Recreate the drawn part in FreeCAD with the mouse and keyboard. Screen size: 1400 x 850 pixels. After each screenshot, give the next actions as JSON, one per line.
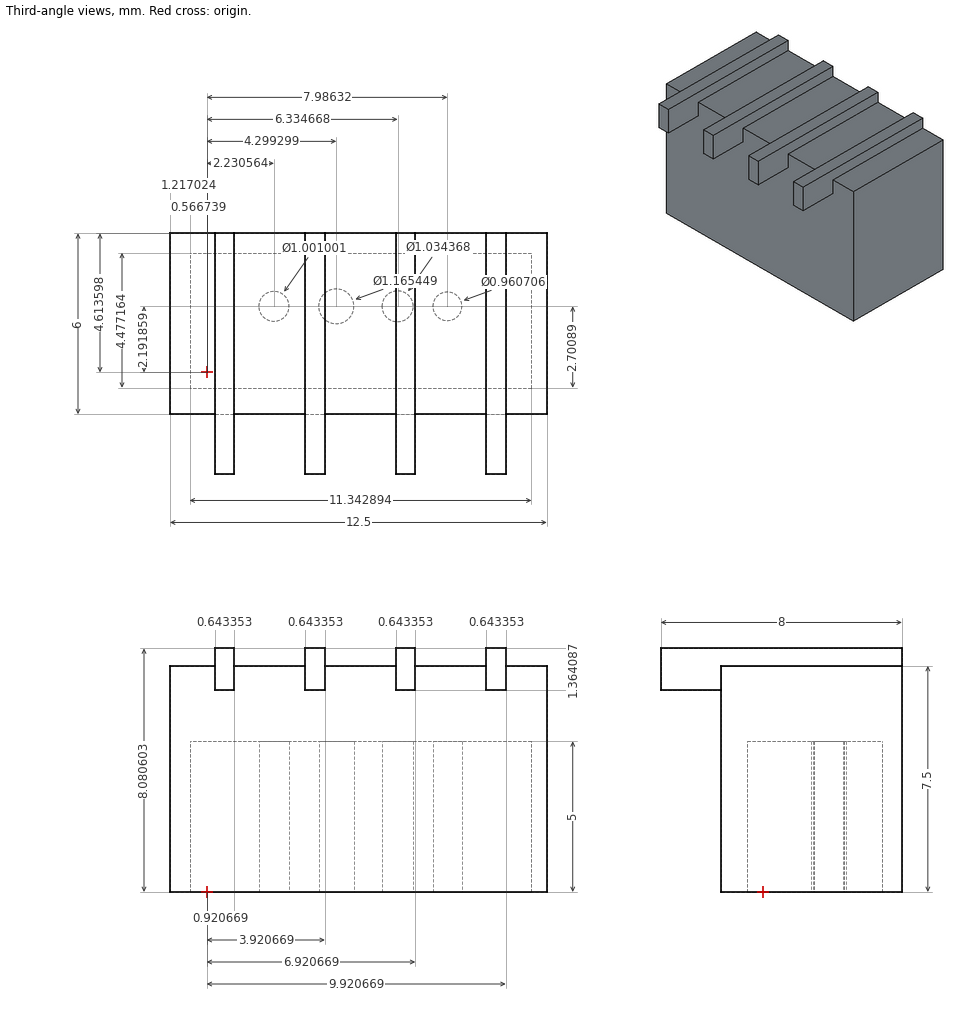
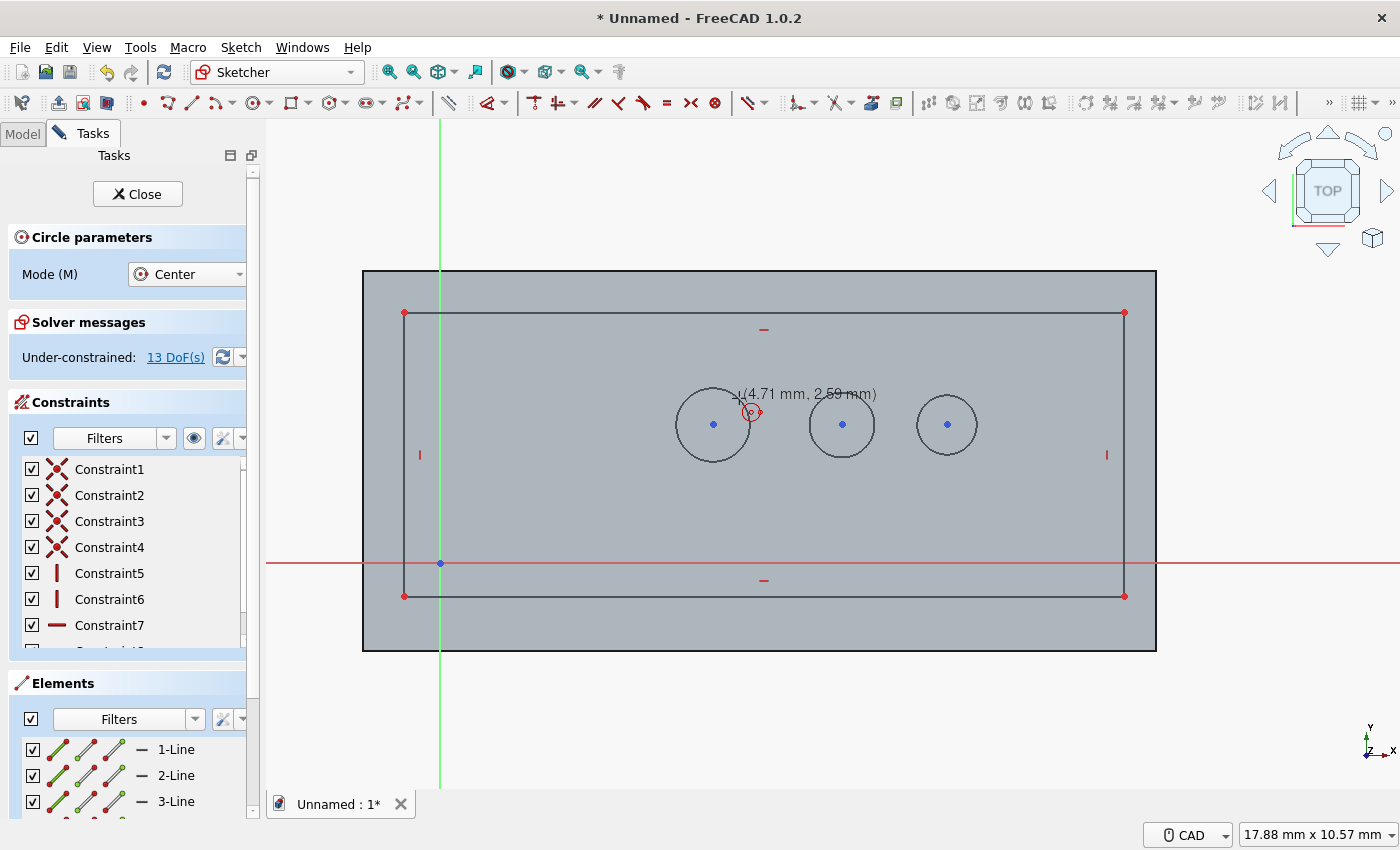
{"action": "left_click", "coordinate": [582, 424]}
{"action": "left_click", "coordinate": [604, 402]}
{"action": "key", "text": "Escape"}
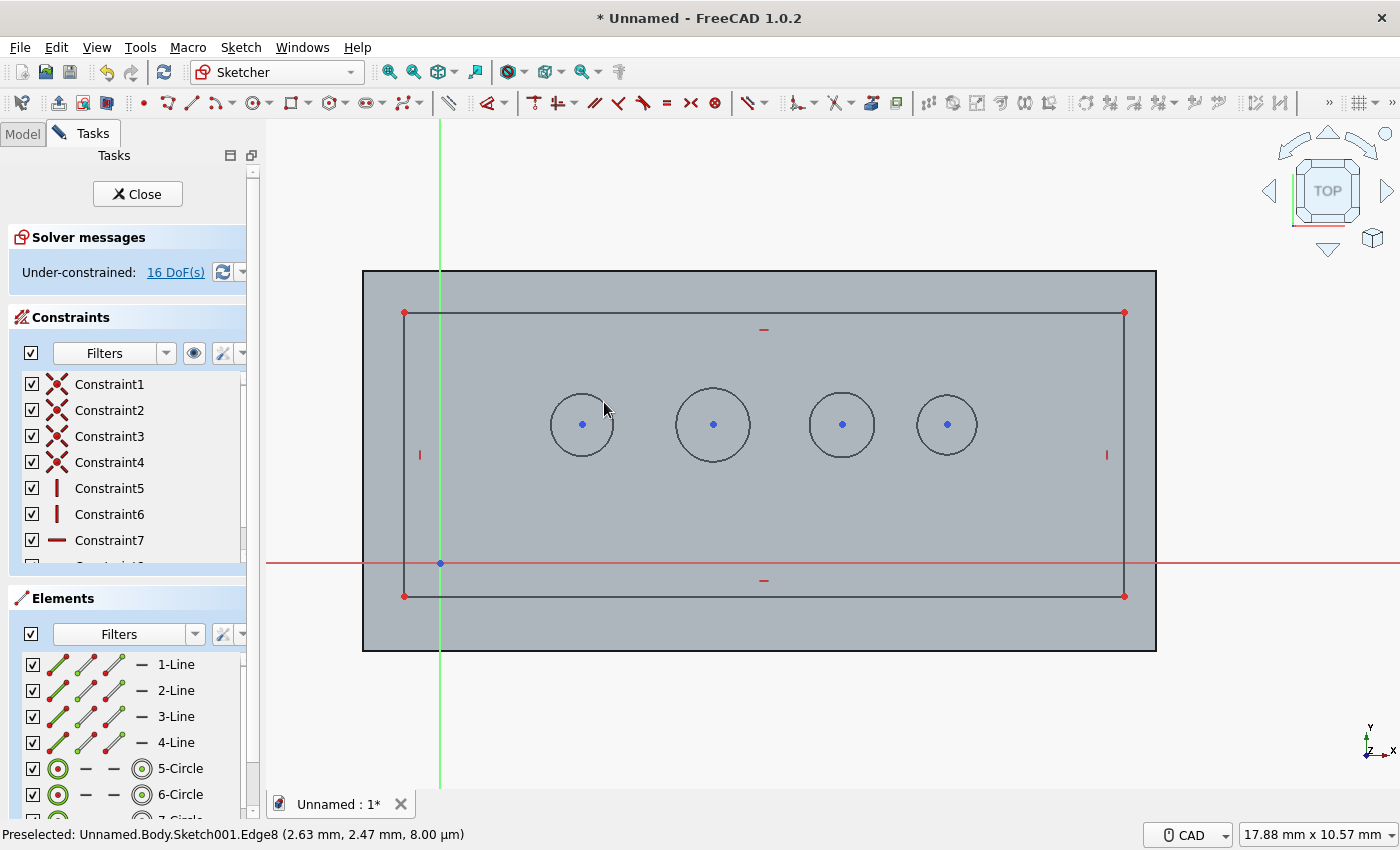
{"action": "left_click", "coordinate": [947, 425]}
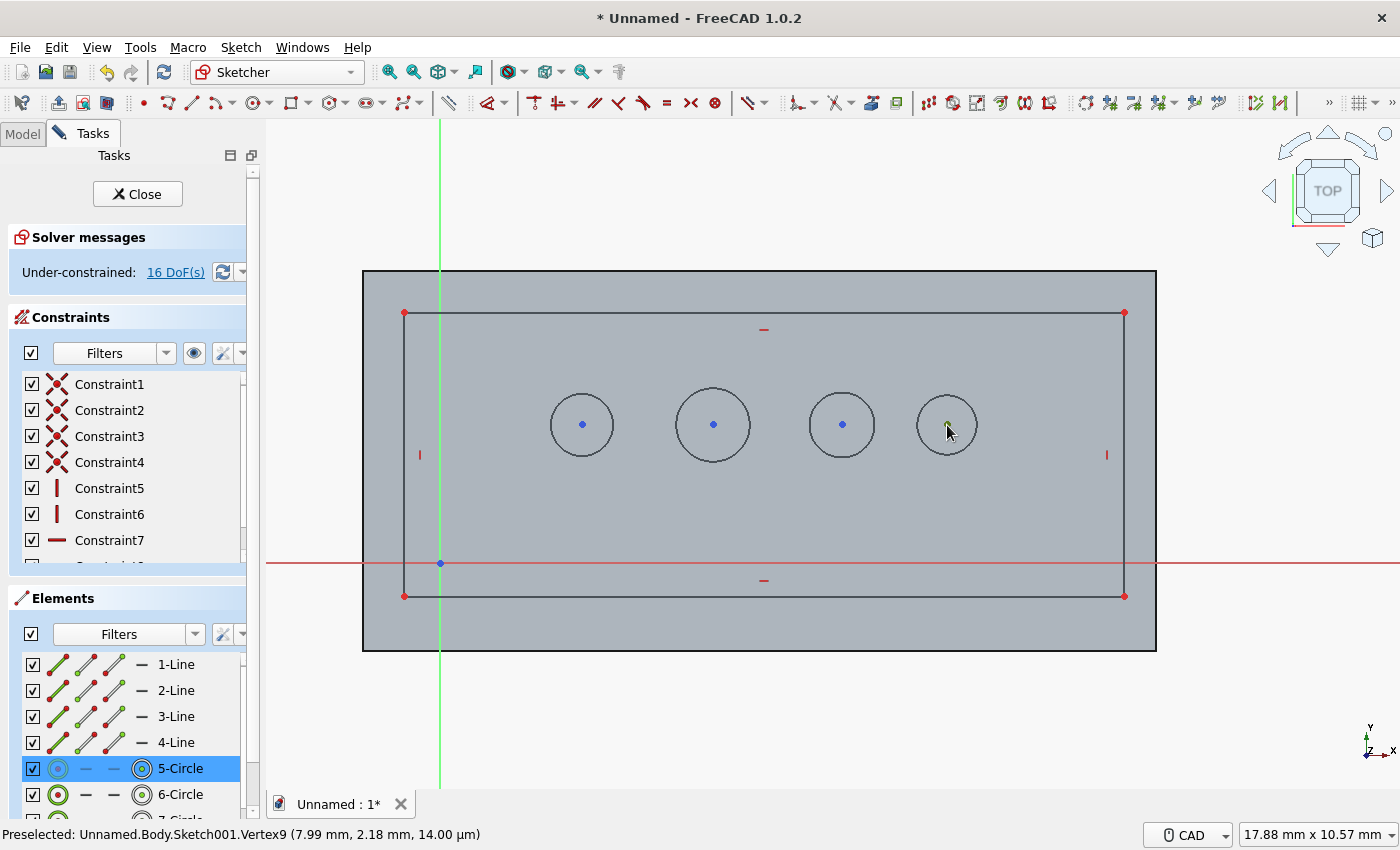
{"action": "left_click", "coordinate": [842, 425]}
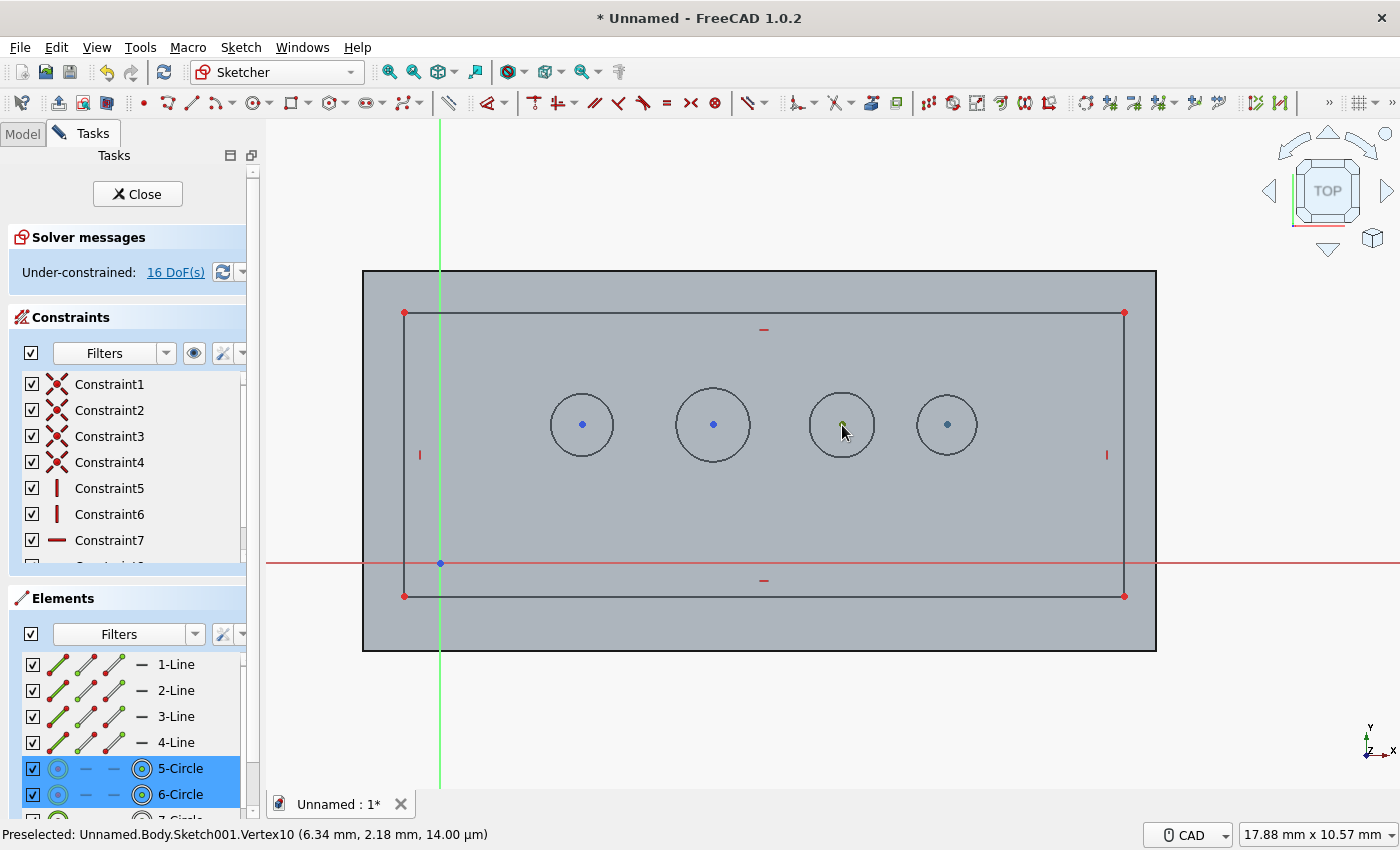
{"action": "key", "text": "h"}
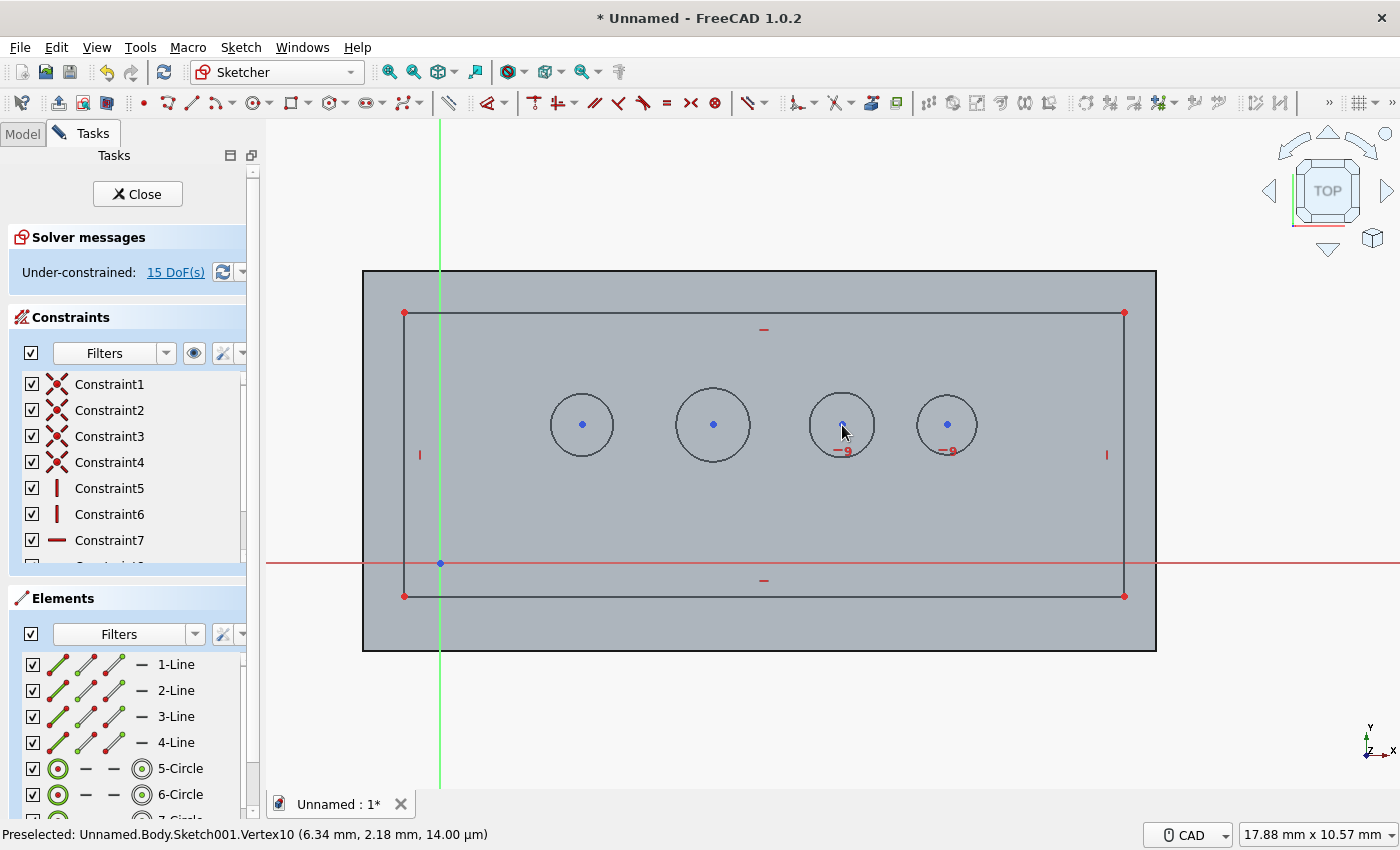
{"action": "left_click", "coordinate": [842, 425]}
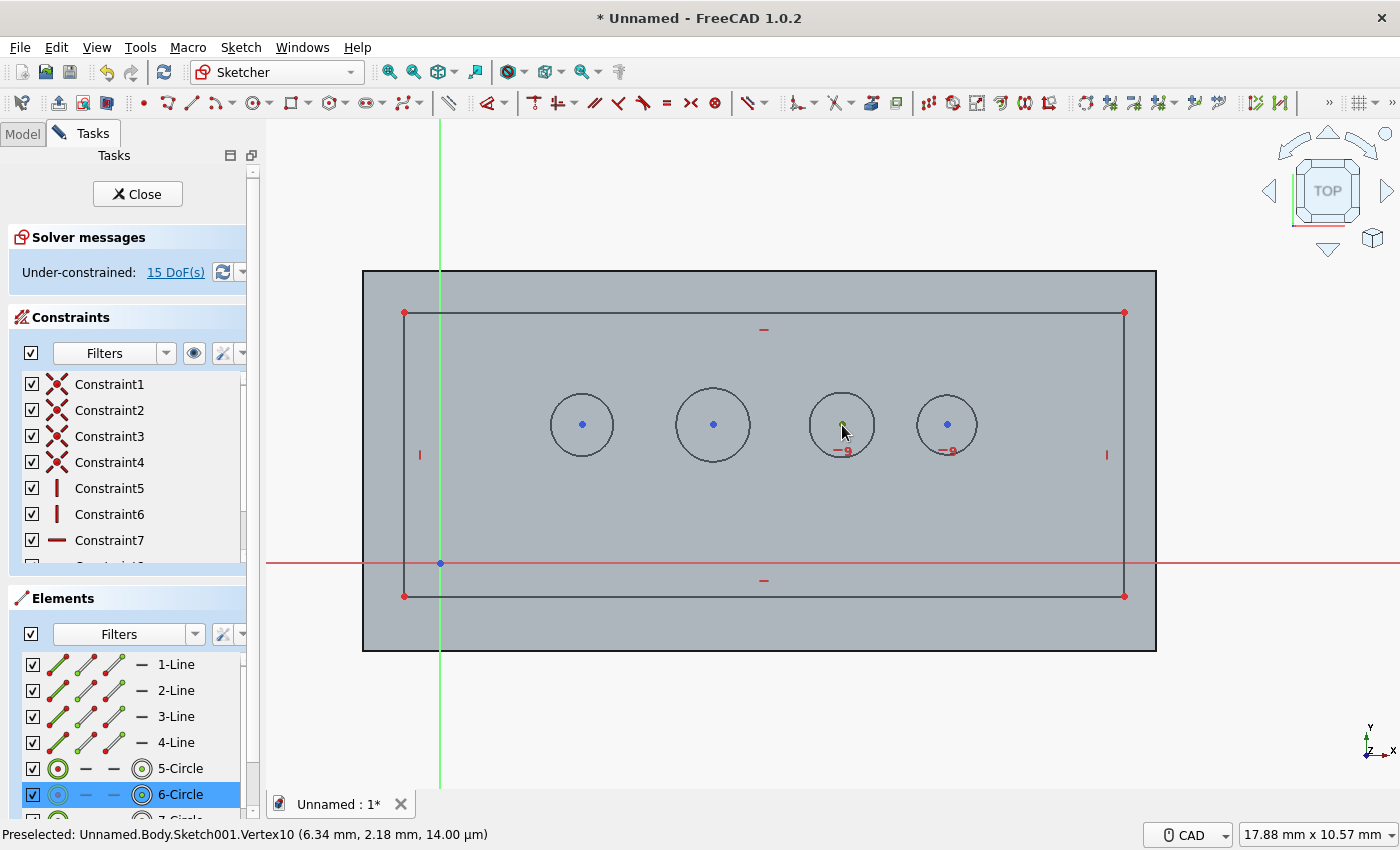
{"action": "left_click", "coordinate": [713, 425]}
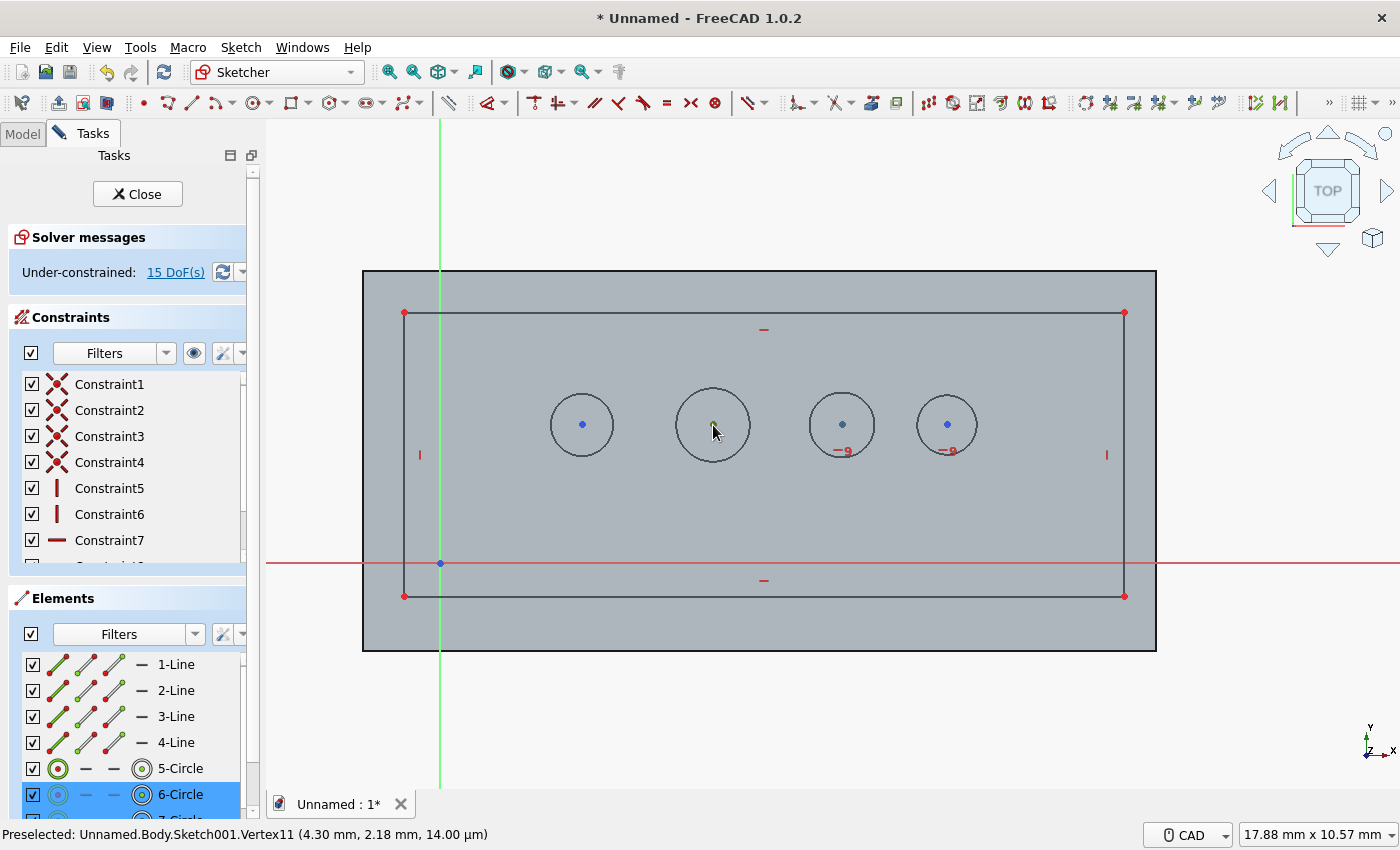
{"action": "key", "text": "h"}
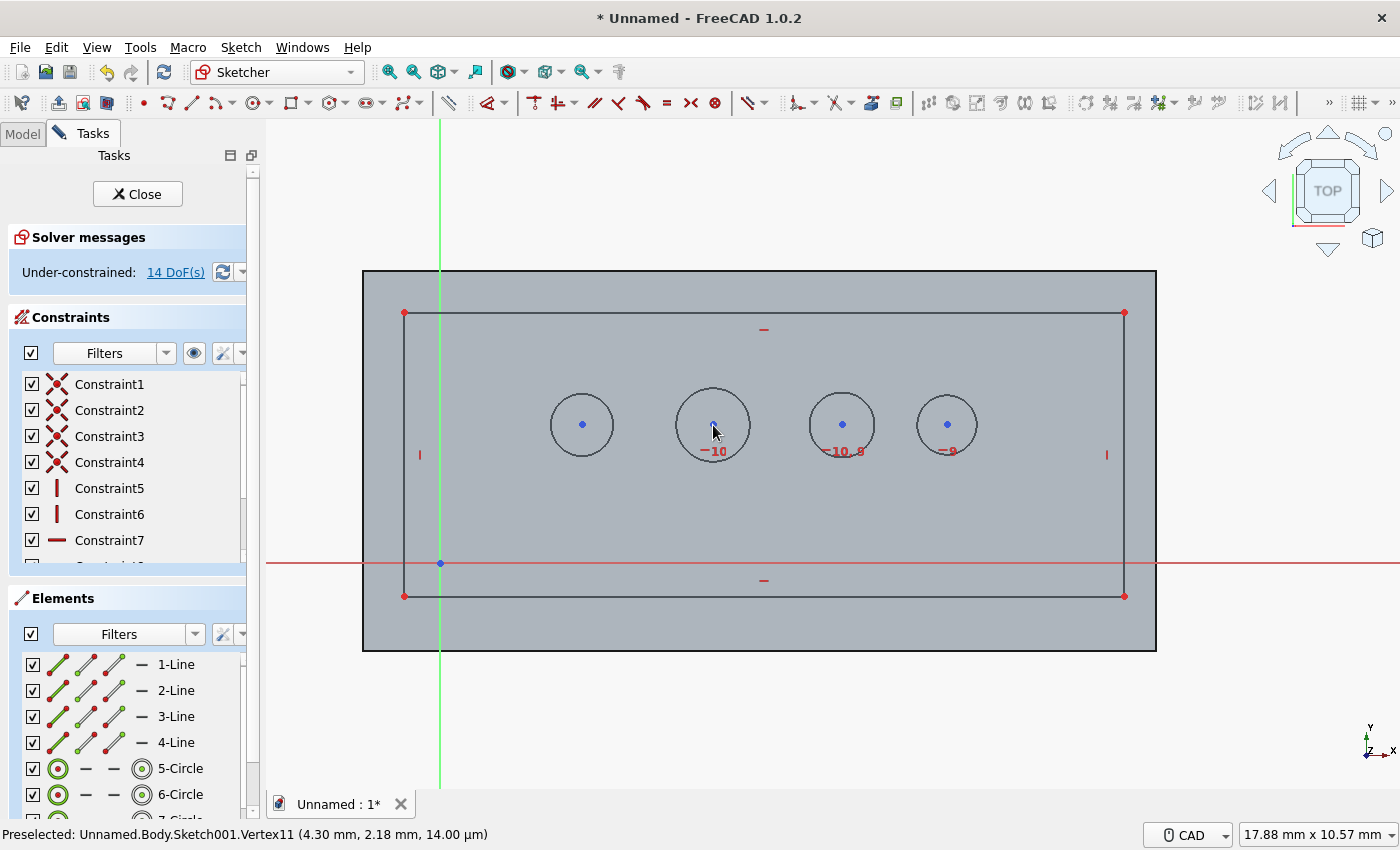
{"action": "left_click", "coordinate": [713, 425]}